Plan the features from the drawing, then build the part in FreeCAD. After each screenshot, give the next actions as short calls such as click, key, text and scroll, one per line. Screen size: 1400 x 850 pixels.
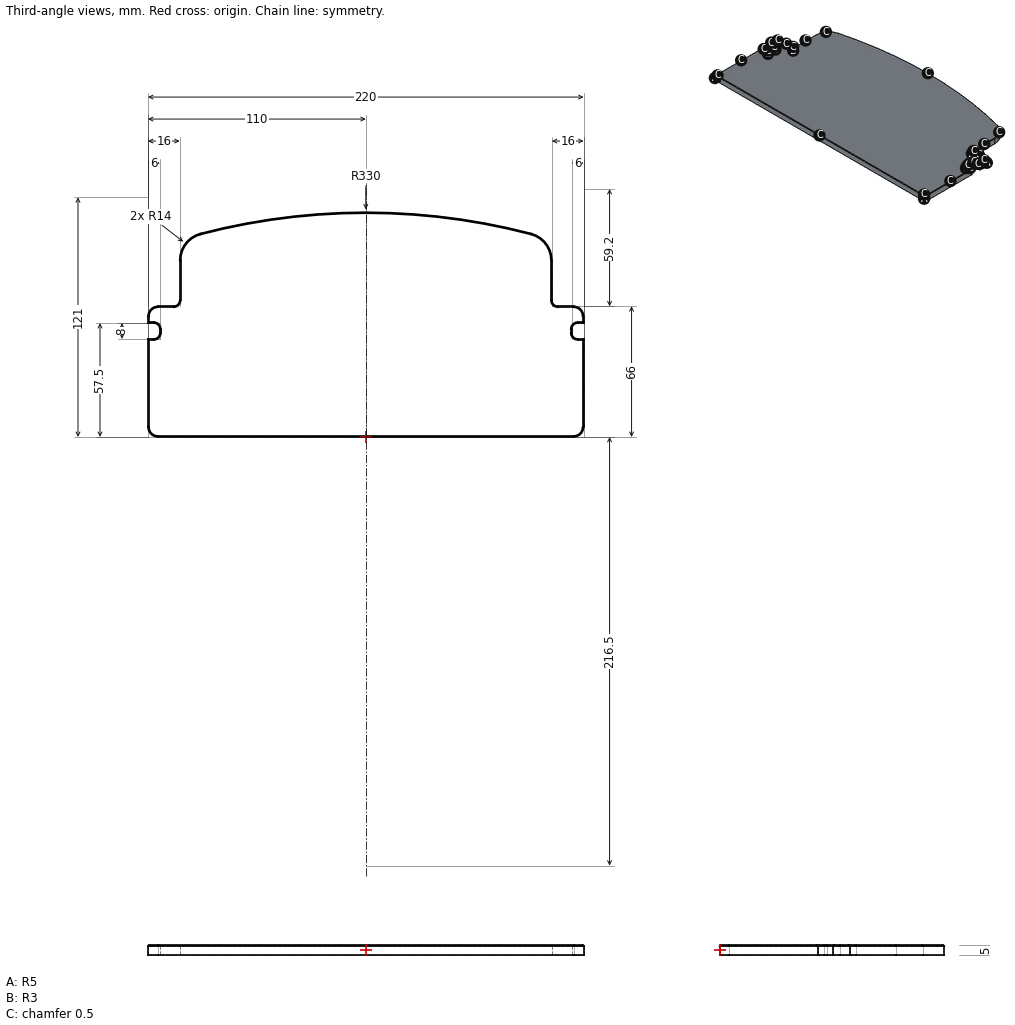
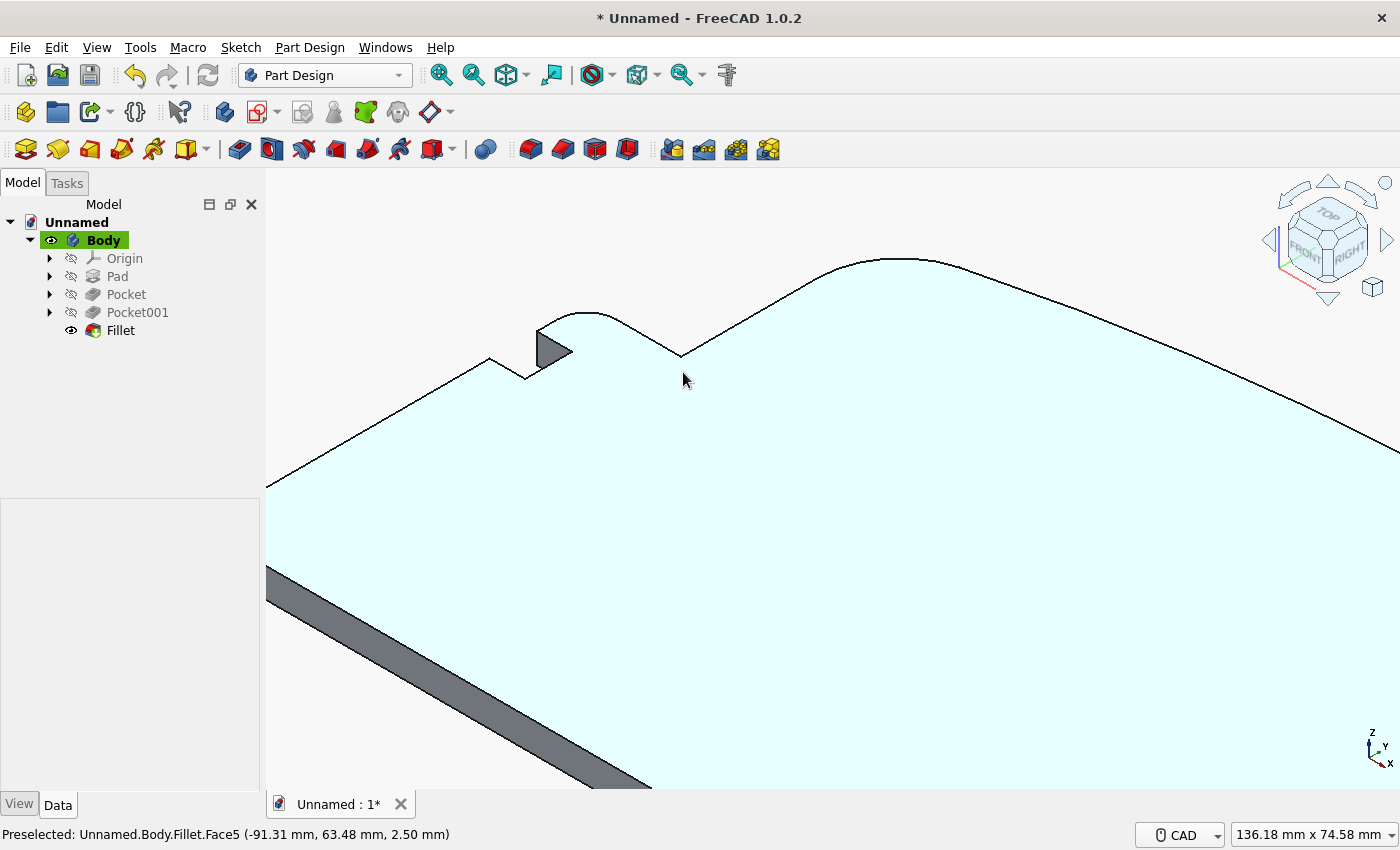
click(442, 76)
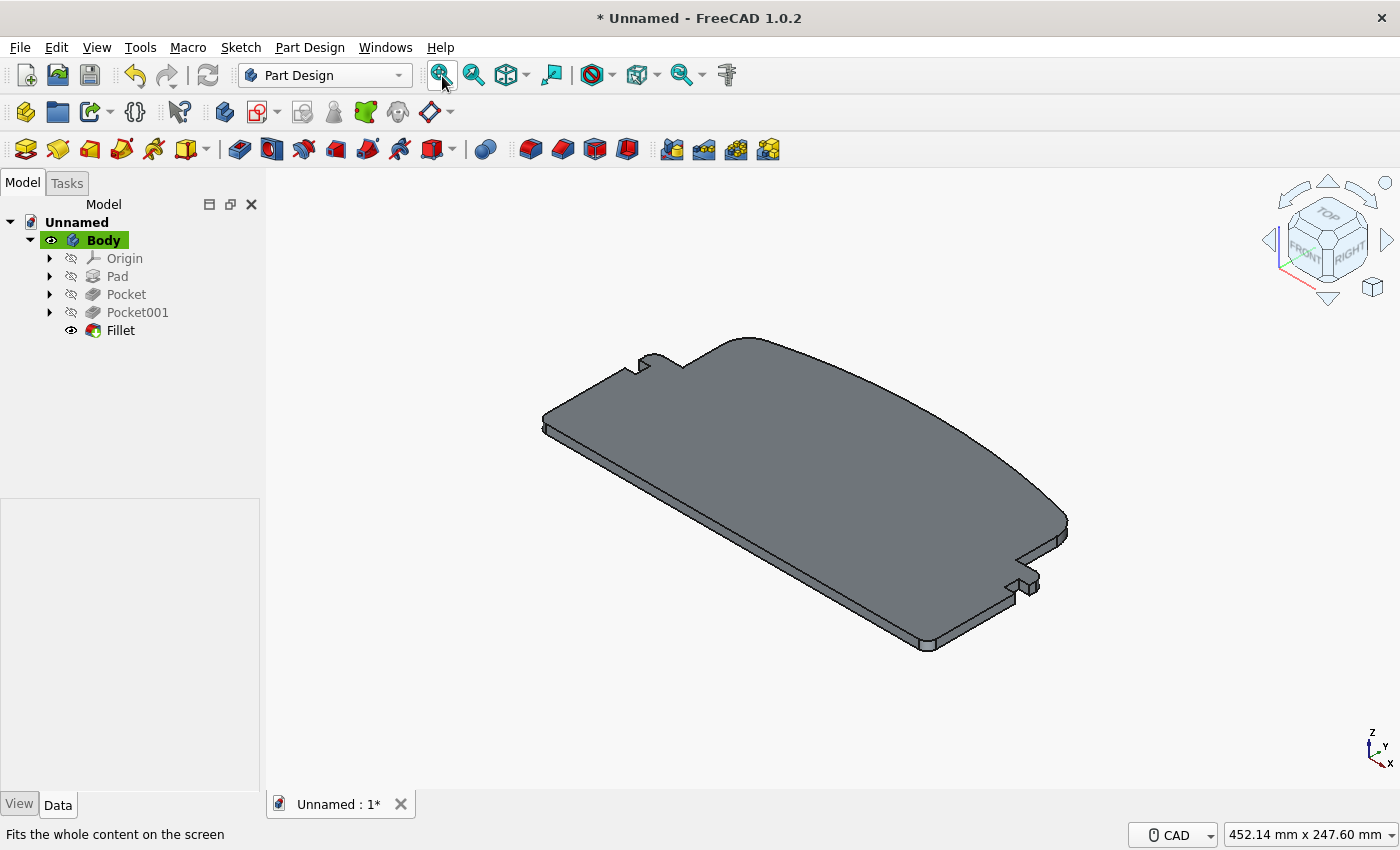
key(2)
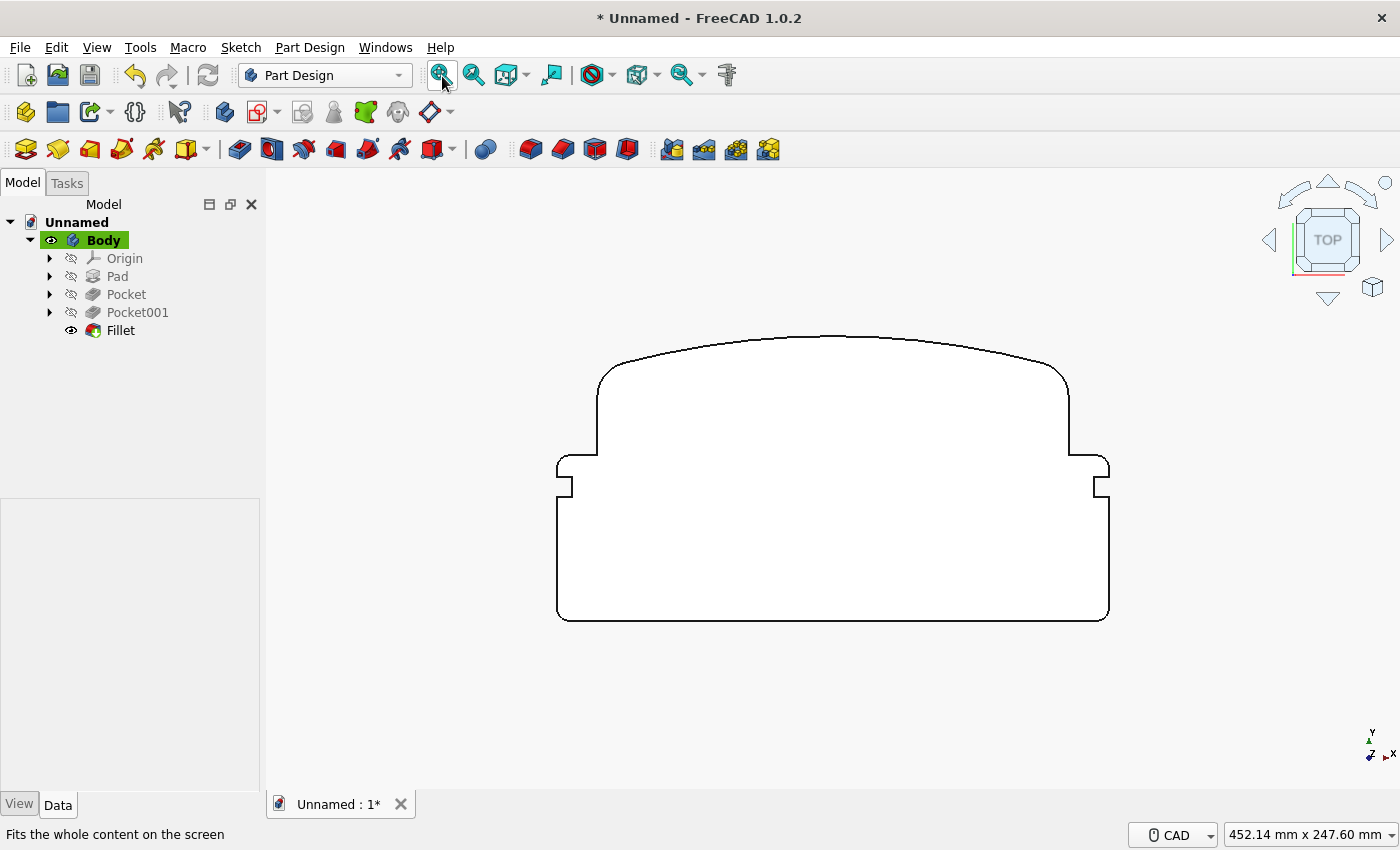
scroll(597, 454, up, 6)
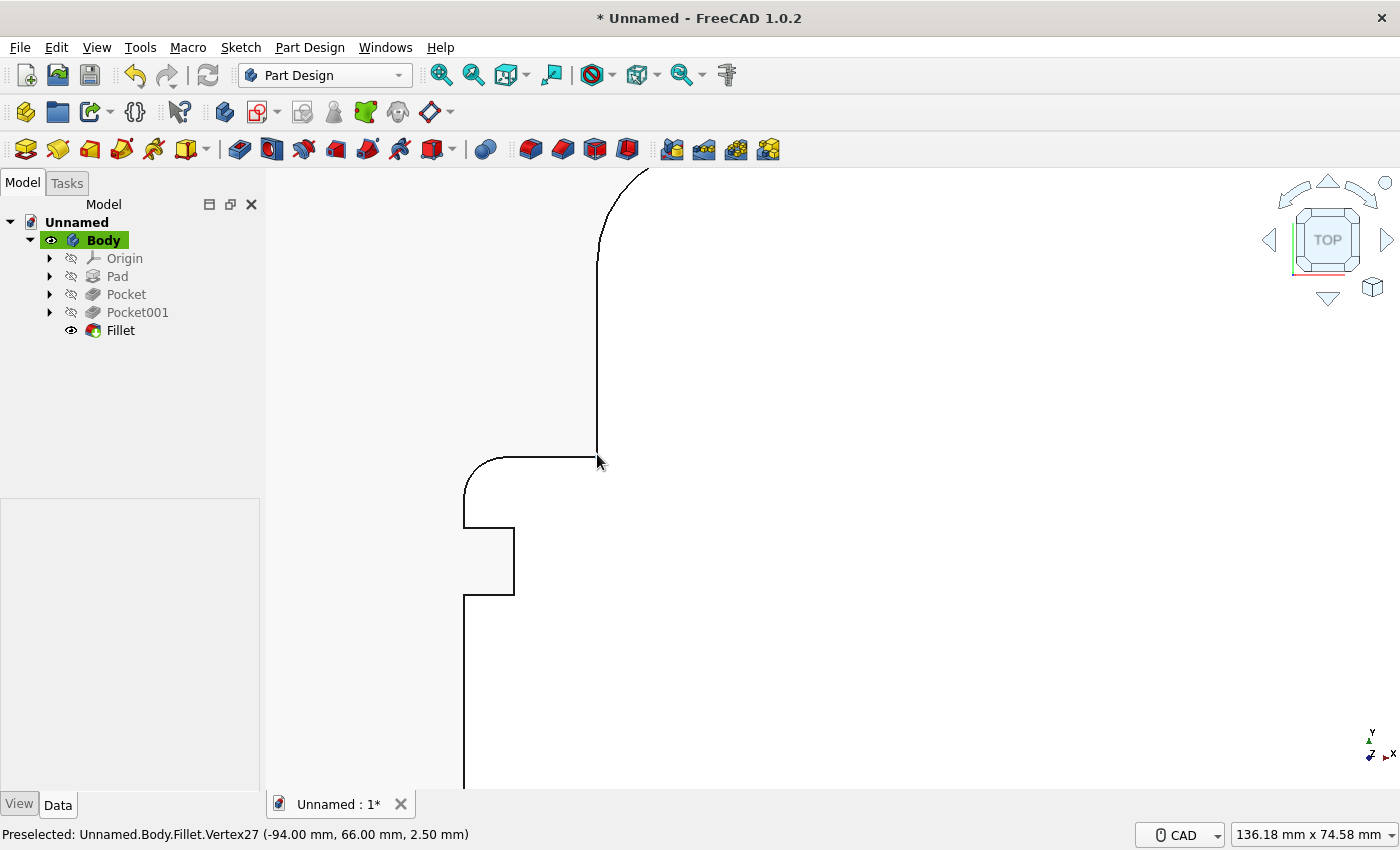
key(v)
key(f)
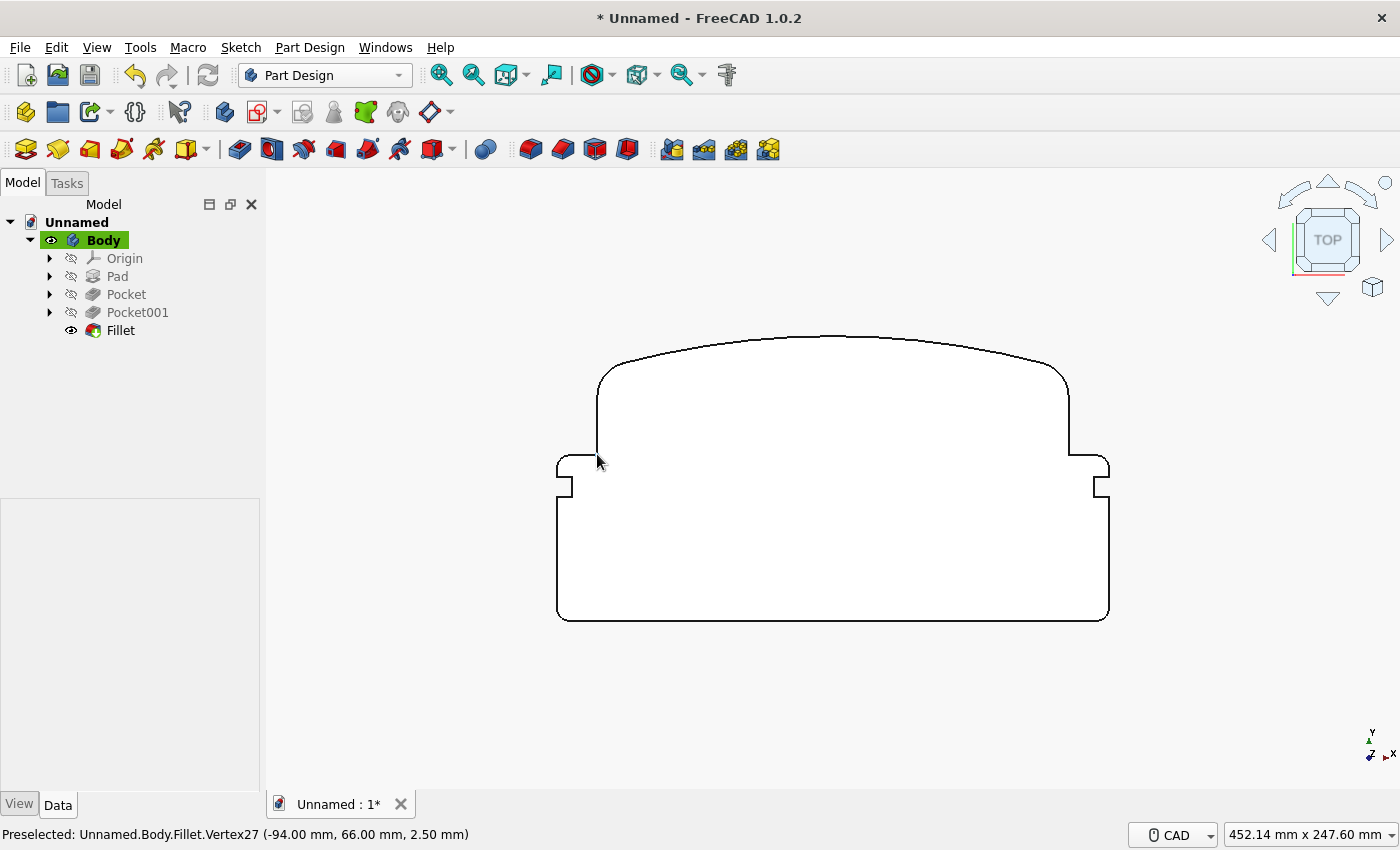
key(1)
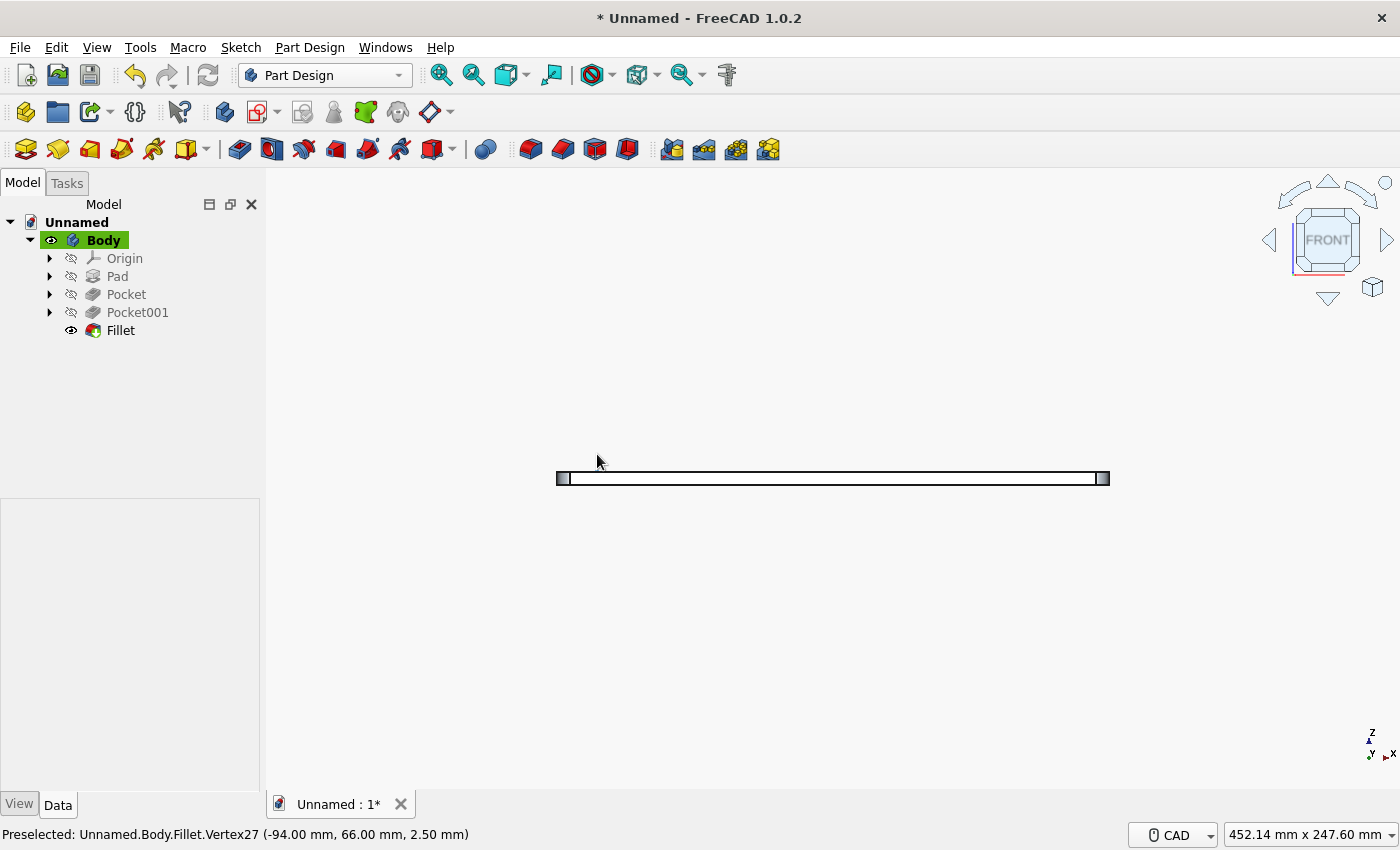
scroll(597, 477, up, 6)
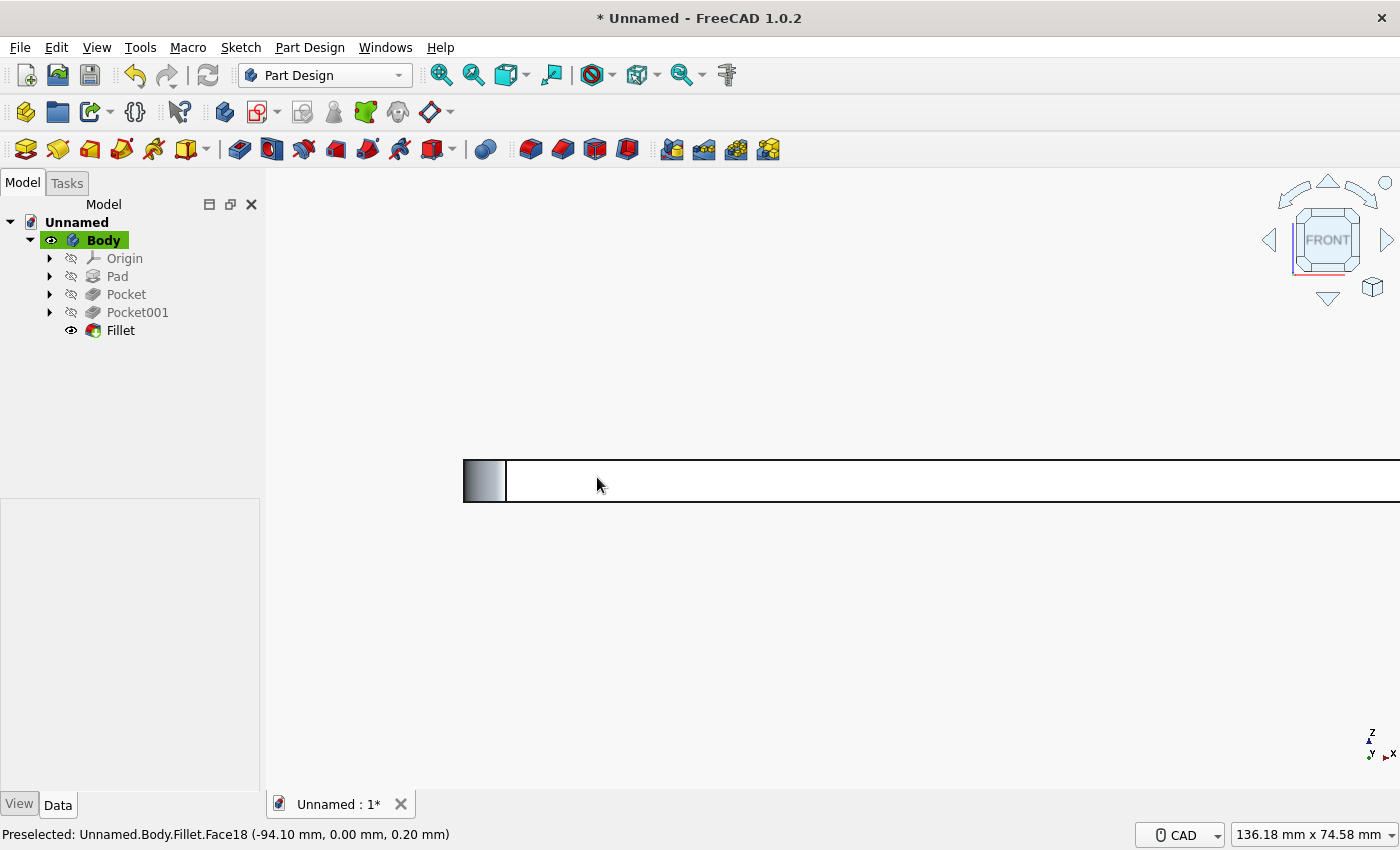
key(v)
key(f)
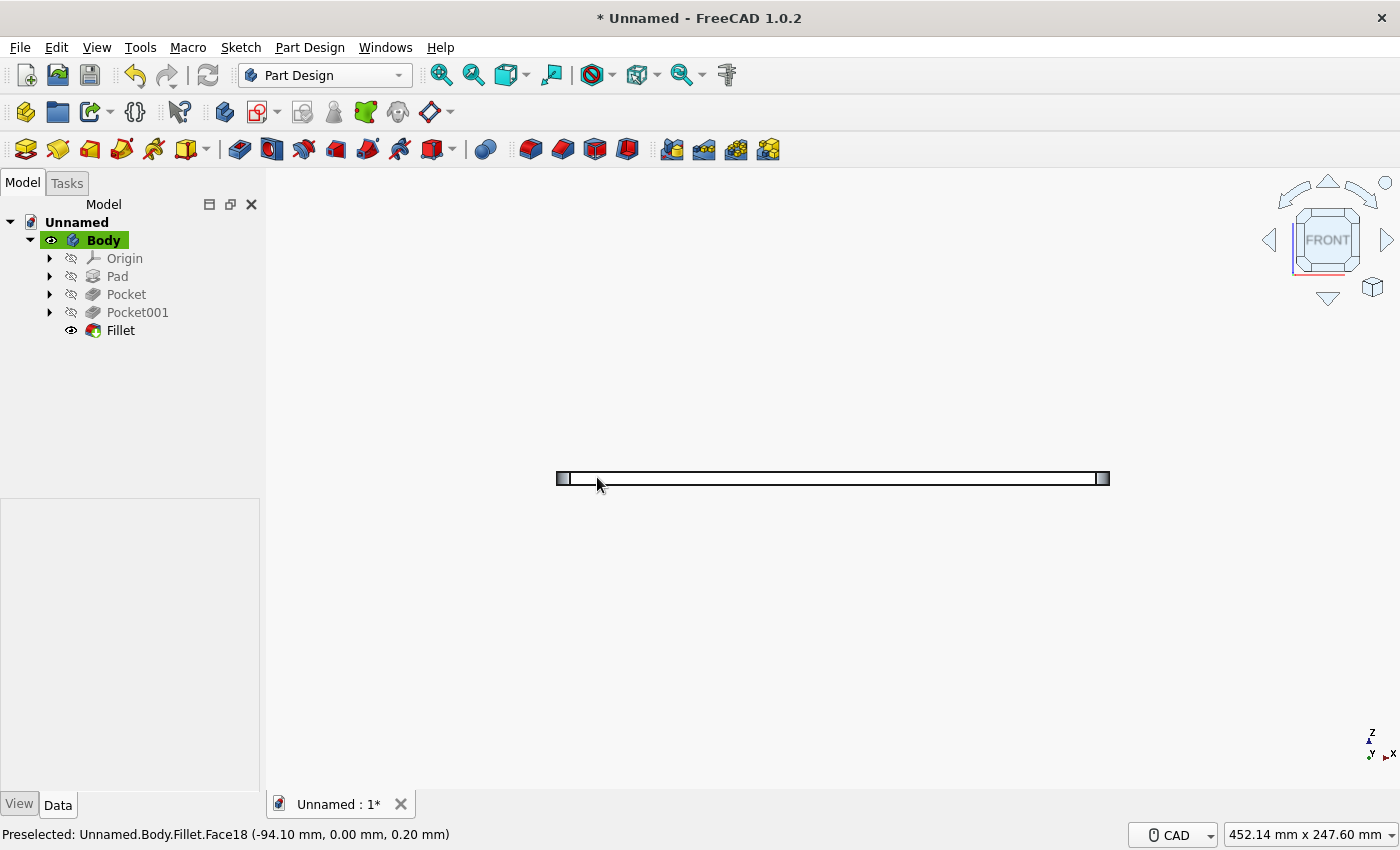
key(3)